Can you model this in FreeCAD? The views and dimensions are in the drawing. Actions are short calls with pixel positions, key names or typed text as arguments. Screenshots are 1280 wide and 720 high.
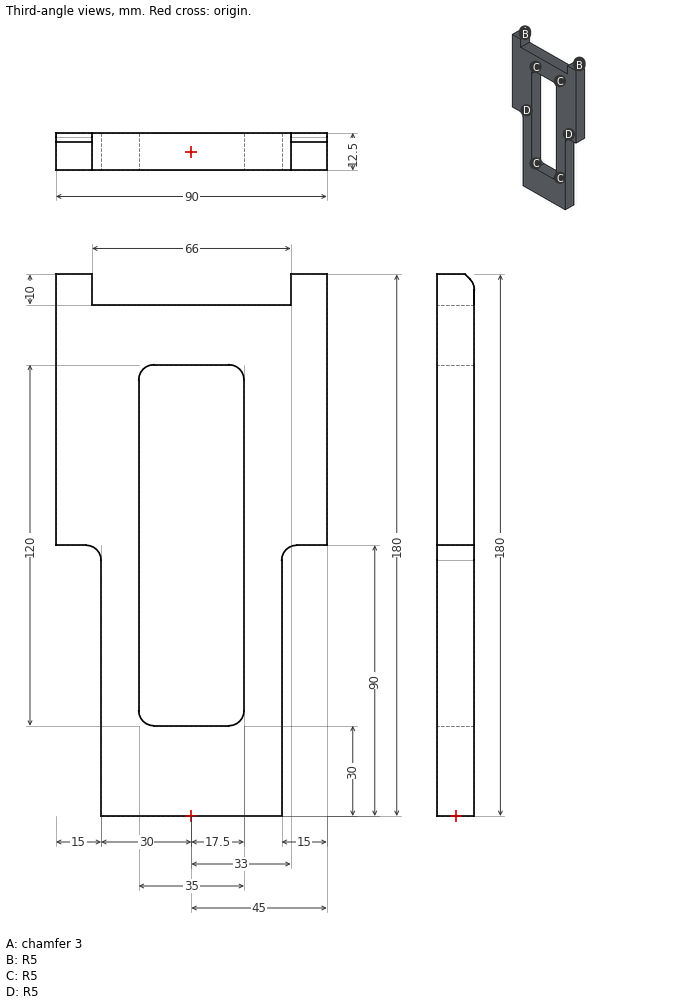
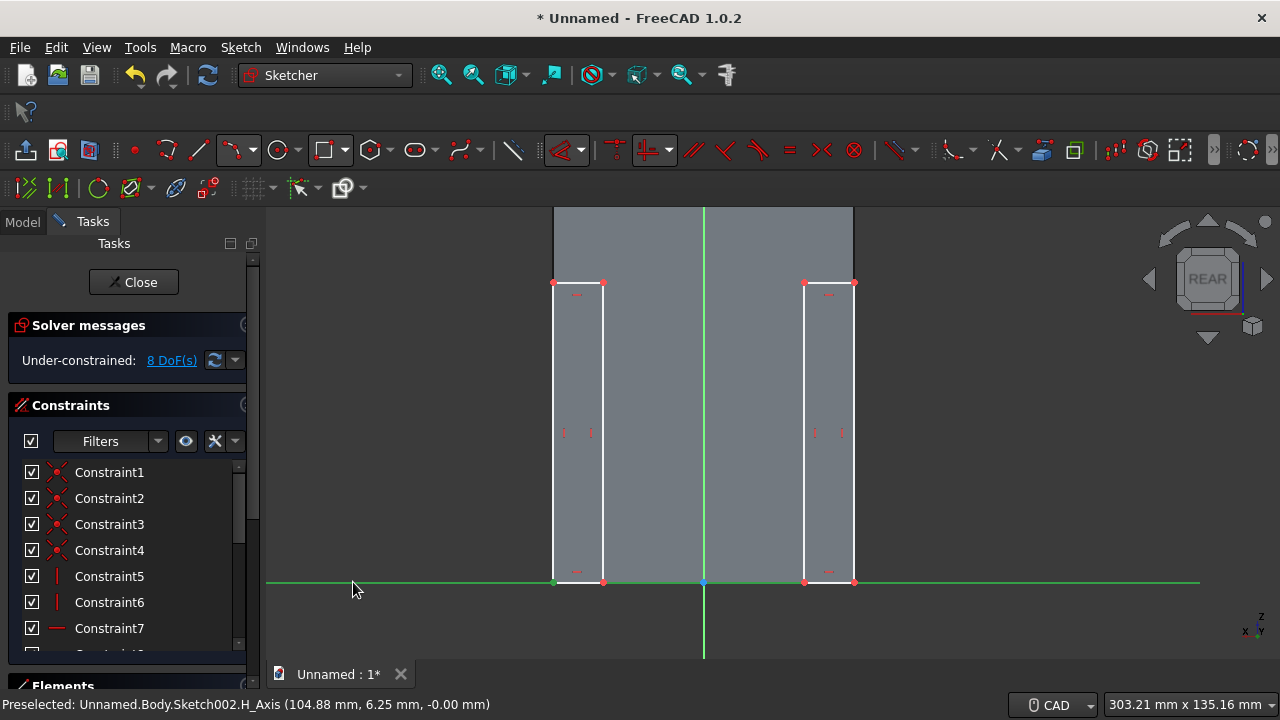
click(616, 150)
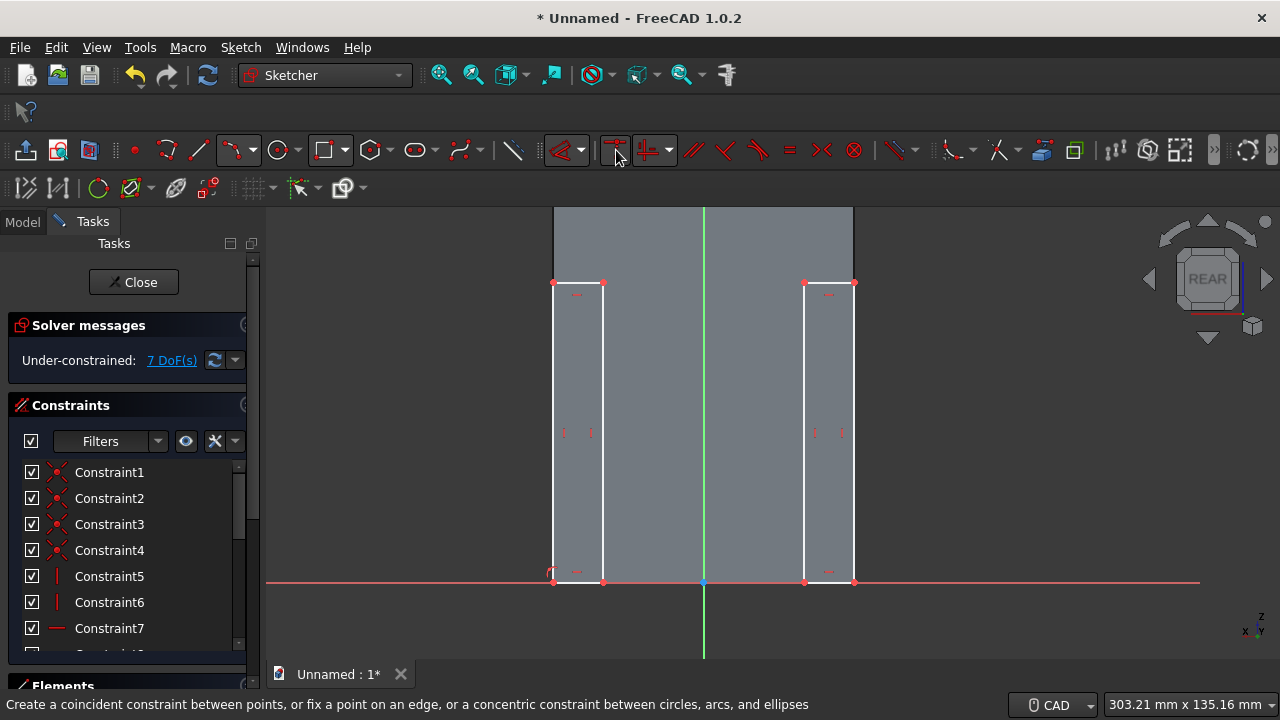
click(804, 583)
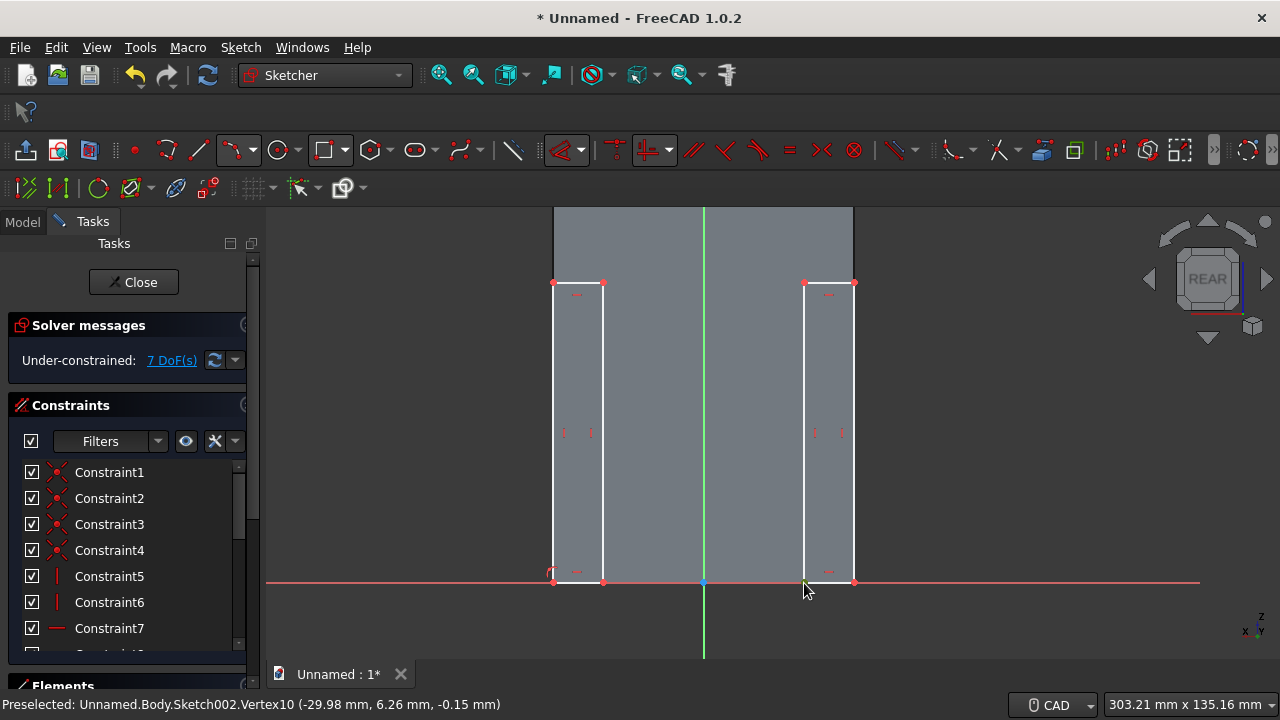
click(353, 582)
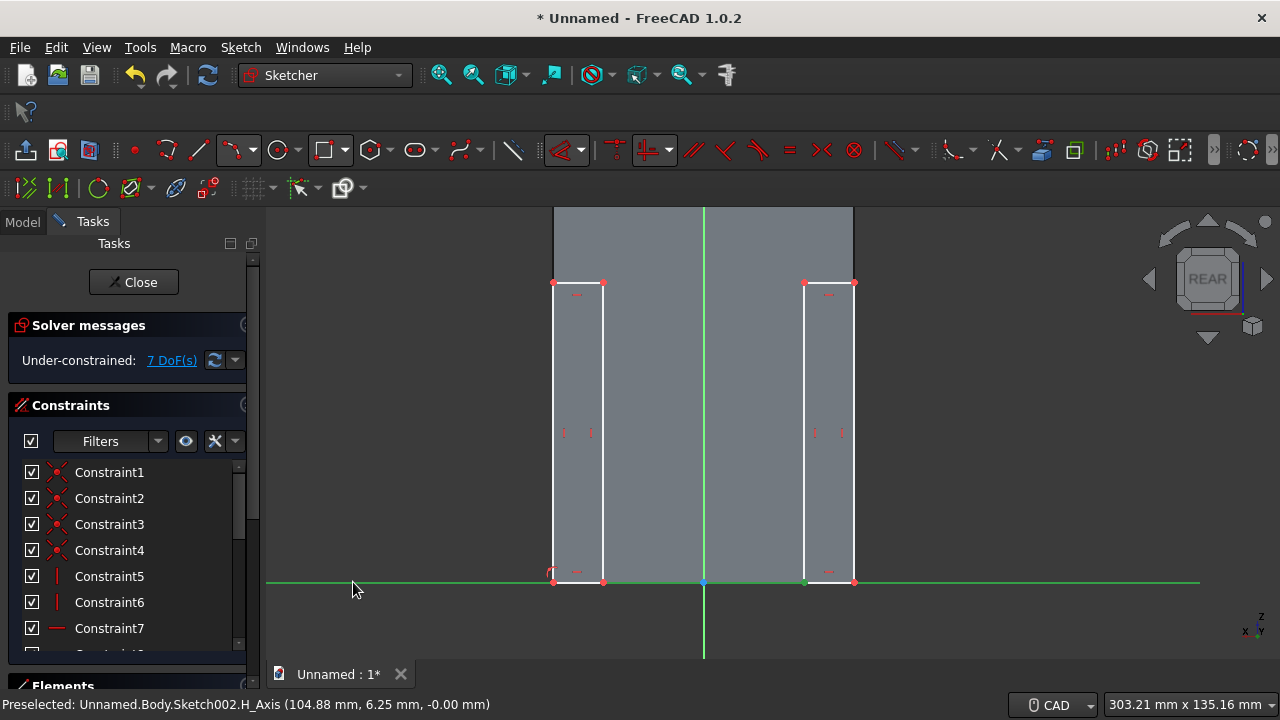
click(616, 150)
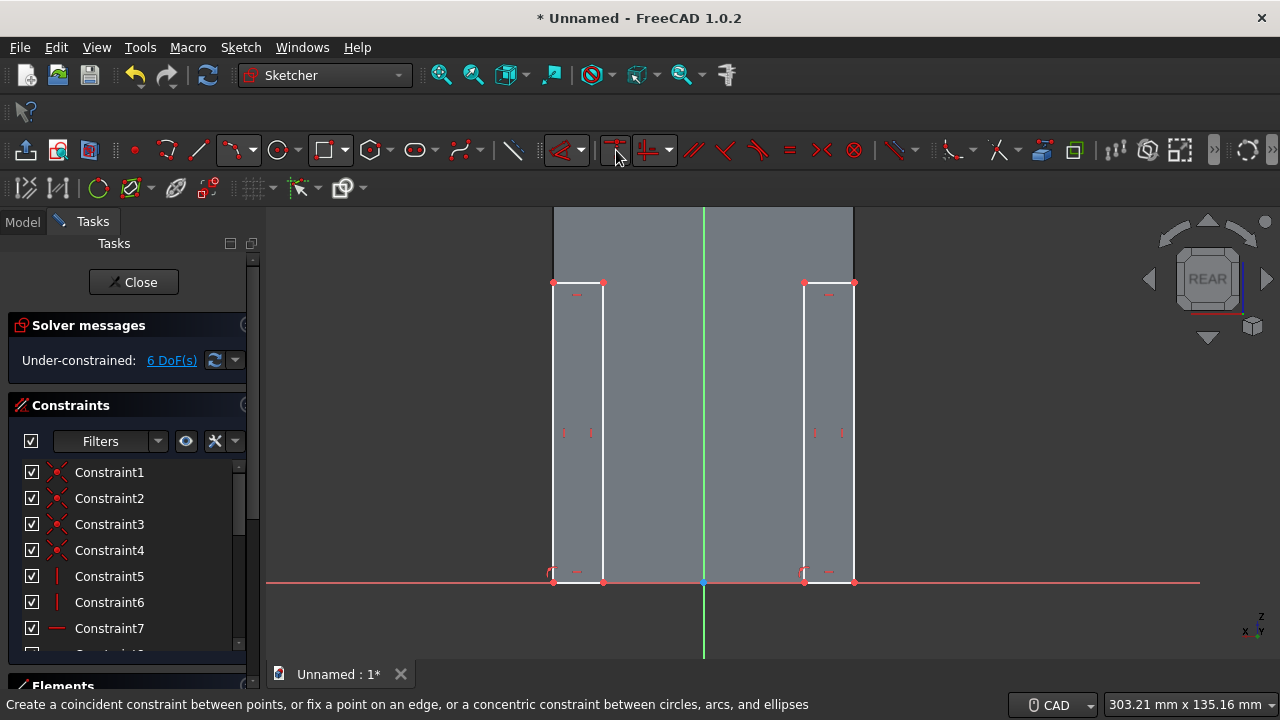
click(553, 373)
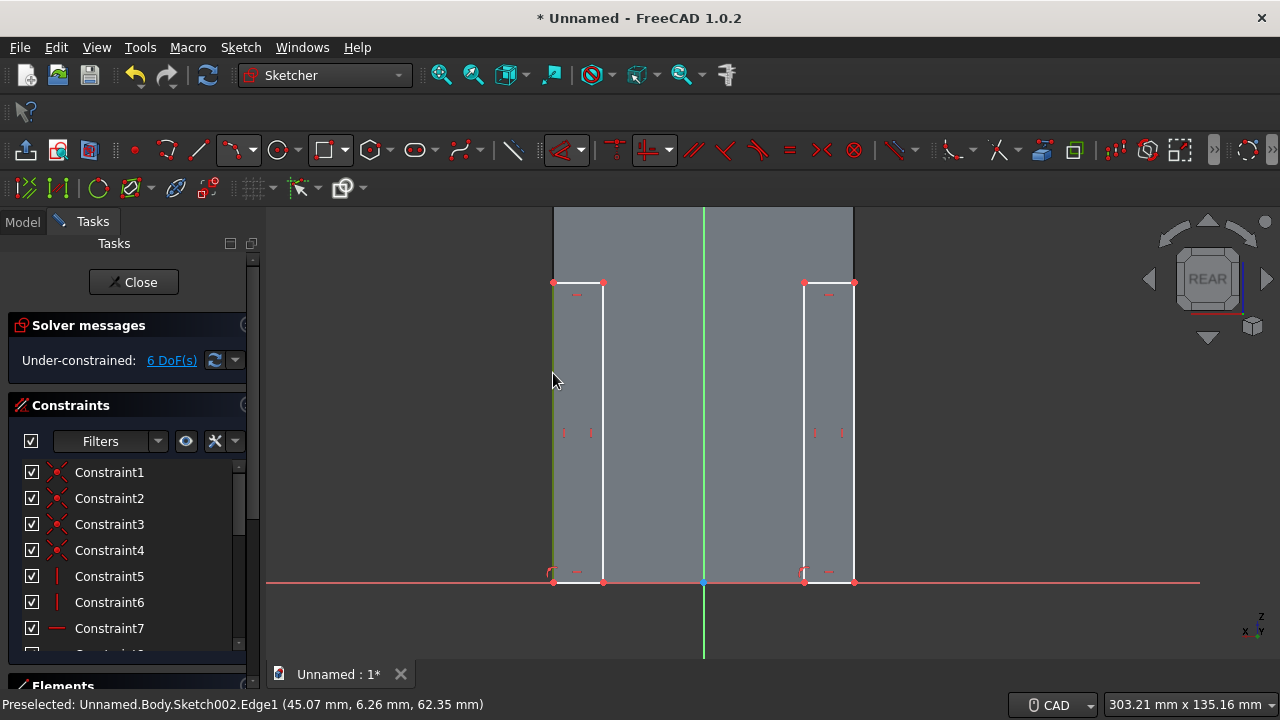
key(i)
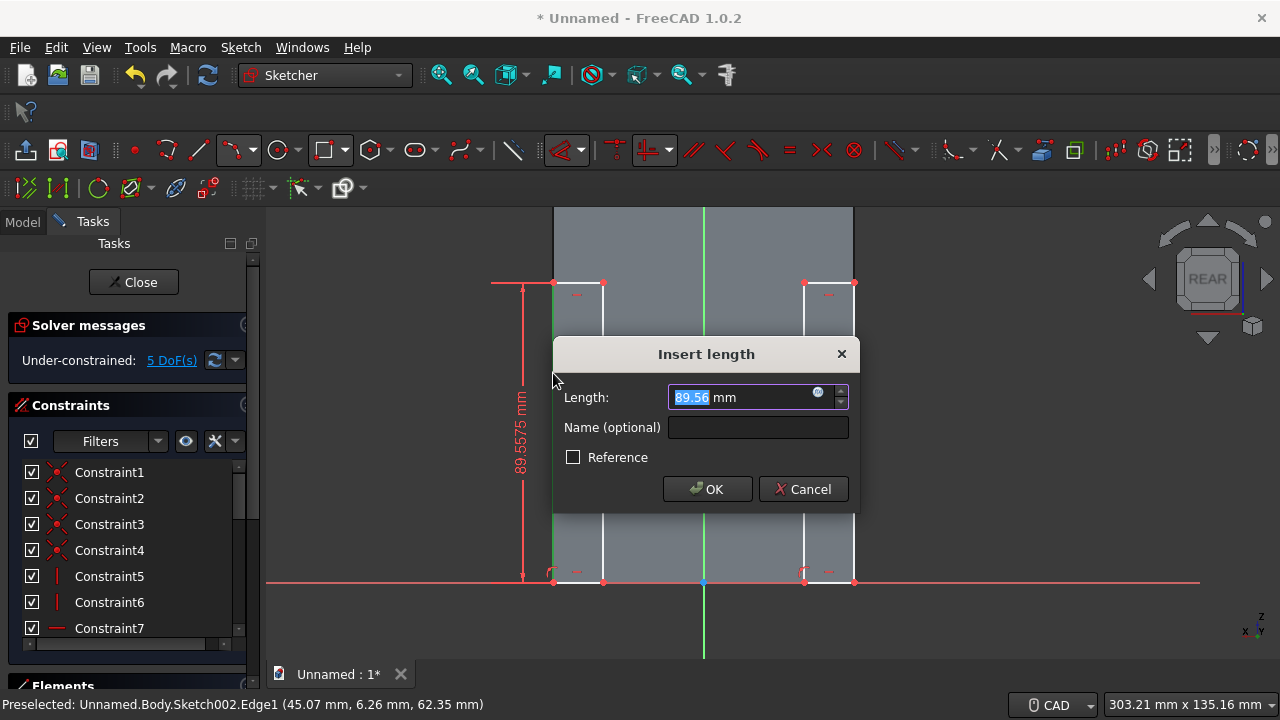
text(90)
key(Return)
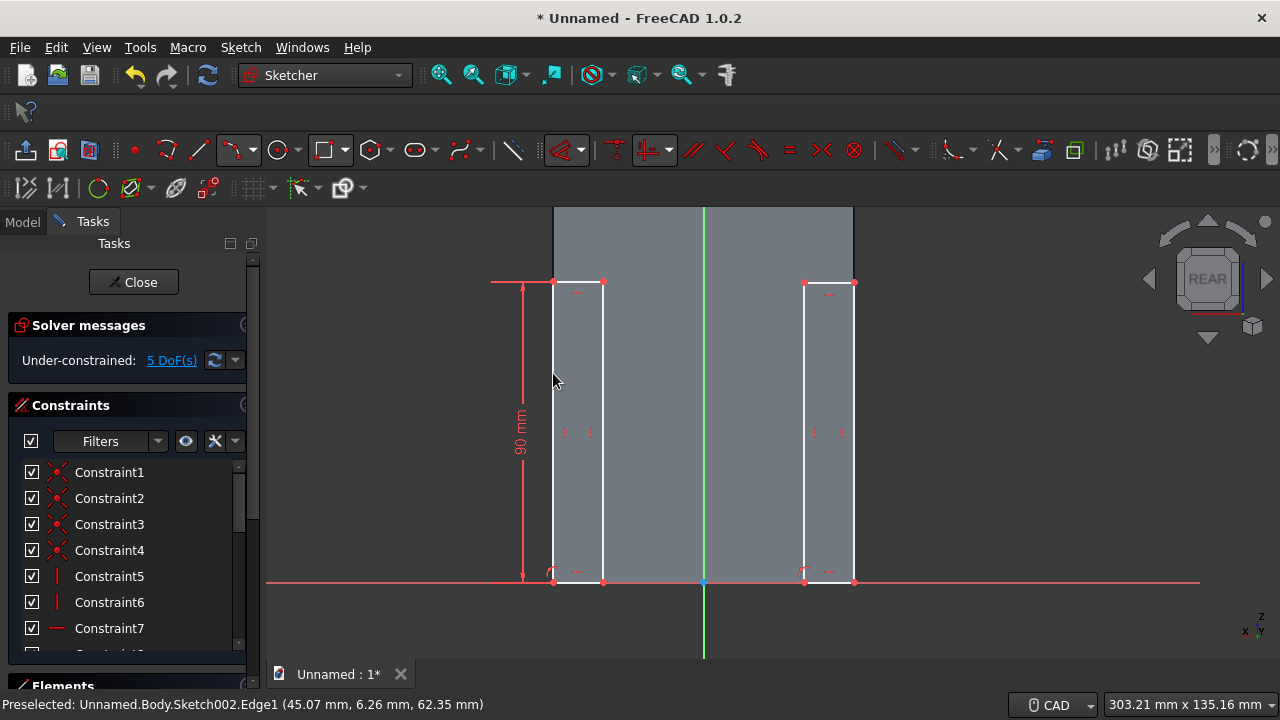
click(568, 582)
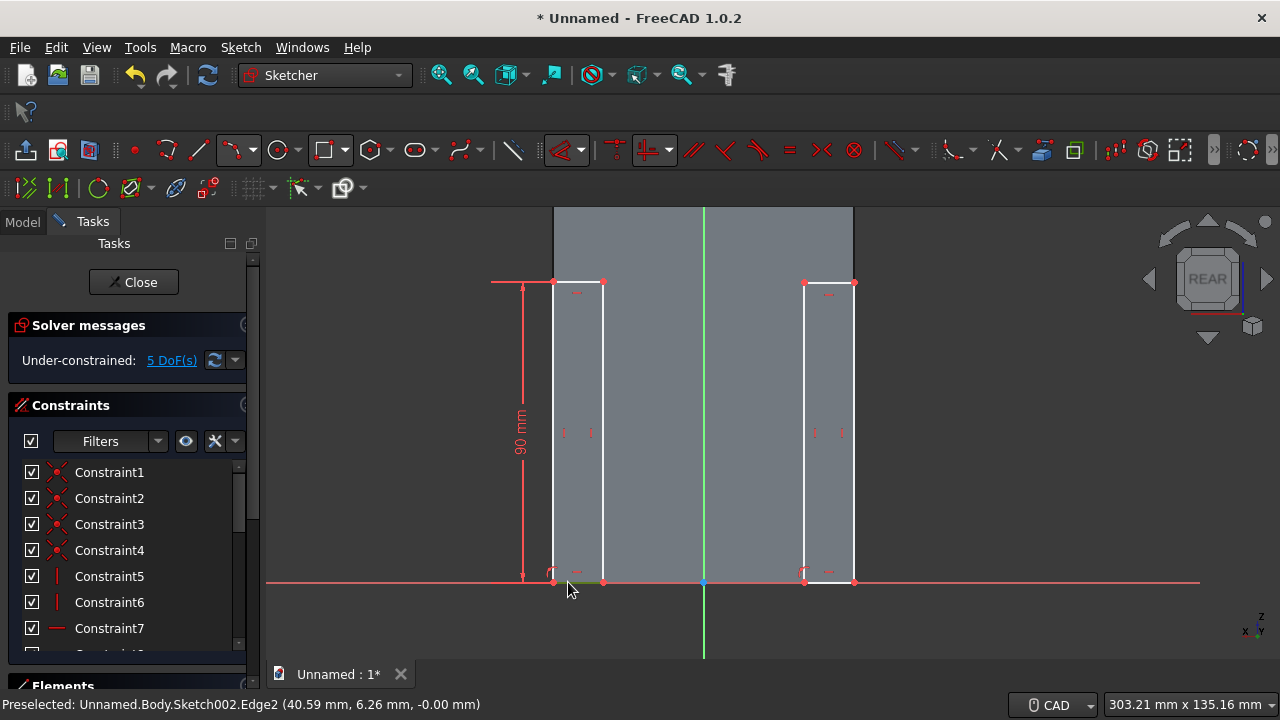
click(584, 150)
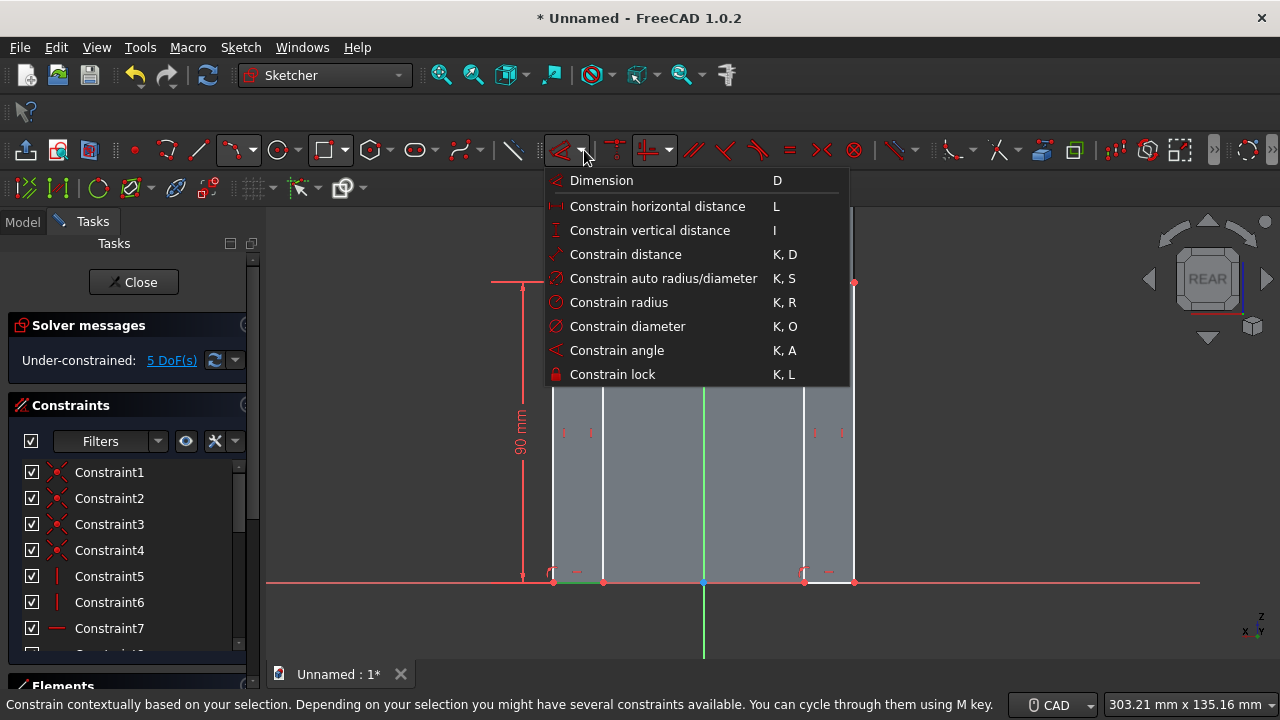
click(697, 206)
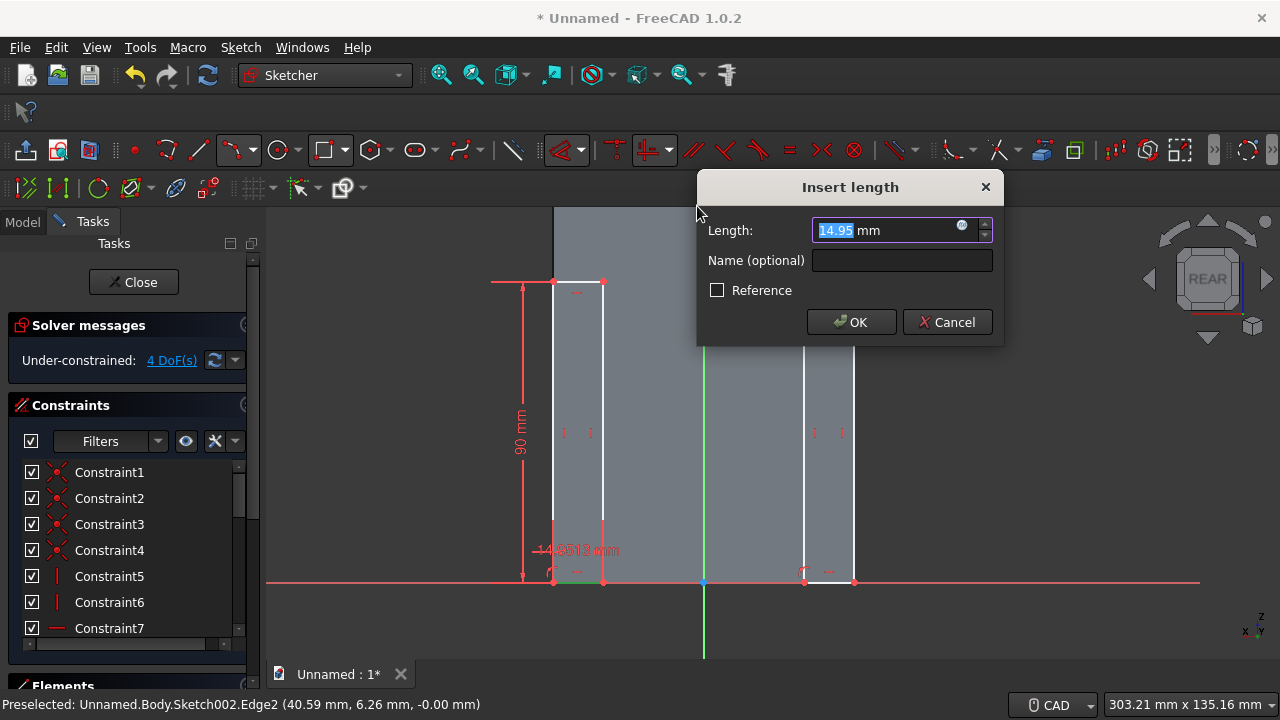
text(15)
key(Return)